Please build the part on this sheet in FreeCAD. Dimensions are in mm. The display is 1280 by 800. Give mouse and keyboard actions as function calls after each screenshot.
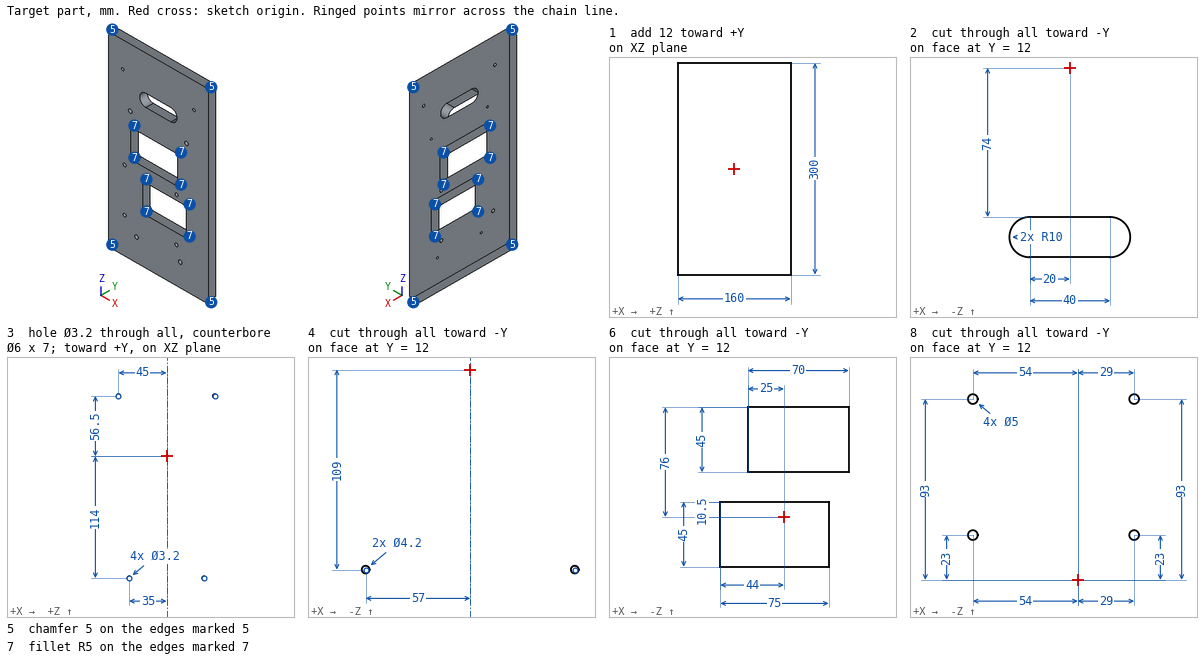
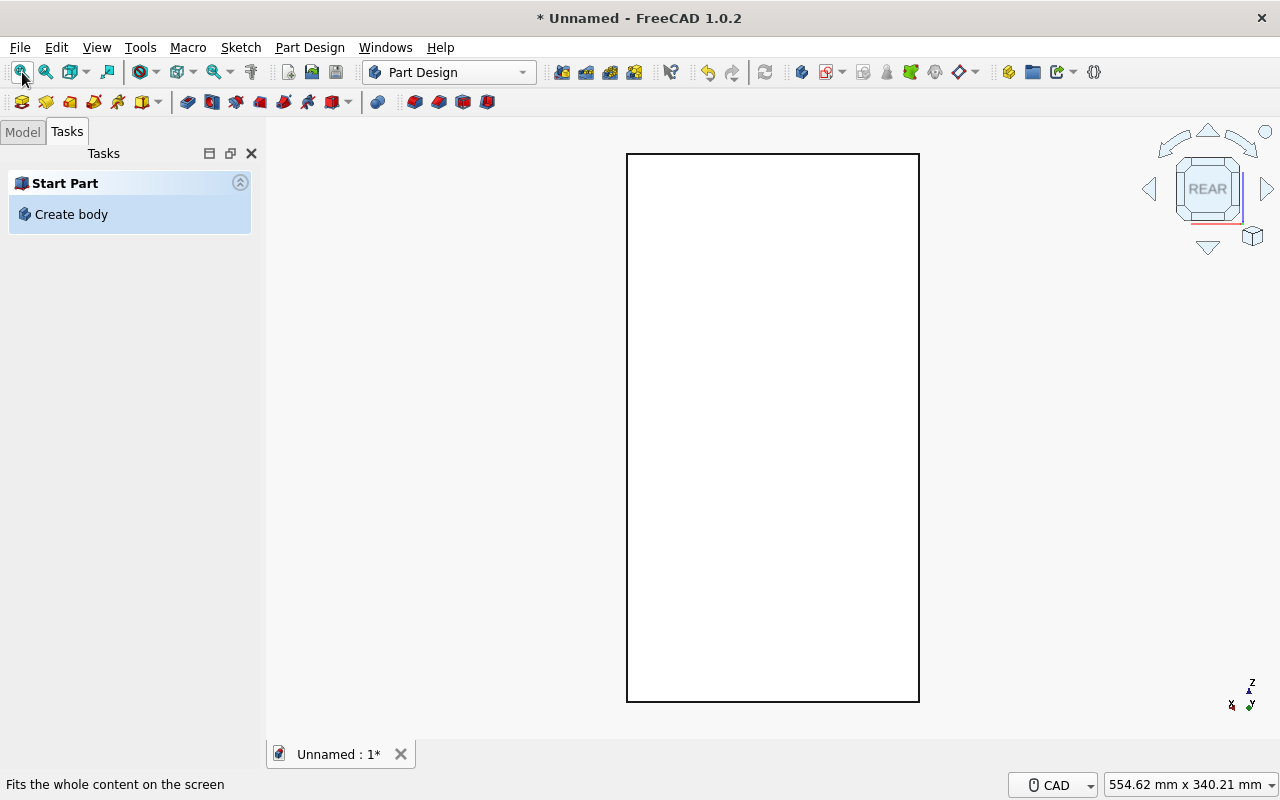
click(773, 349)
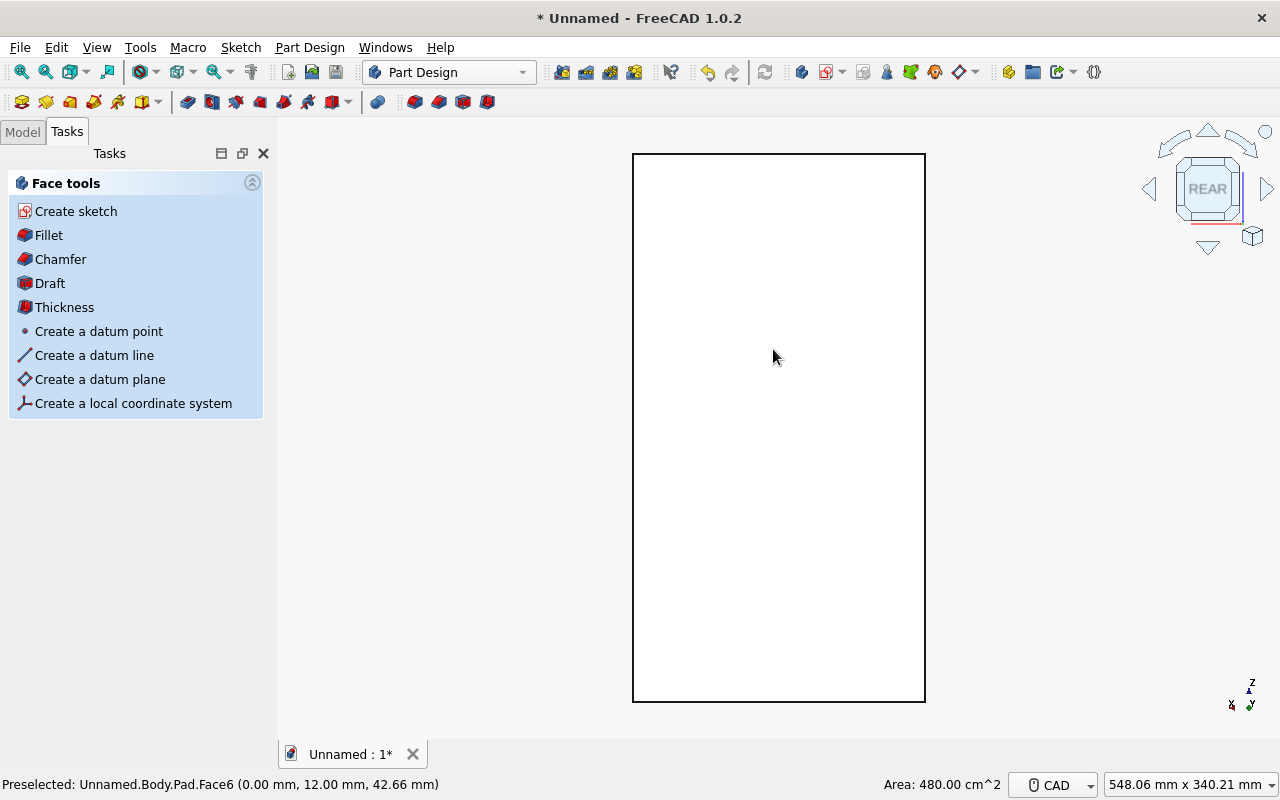
click(826, 72)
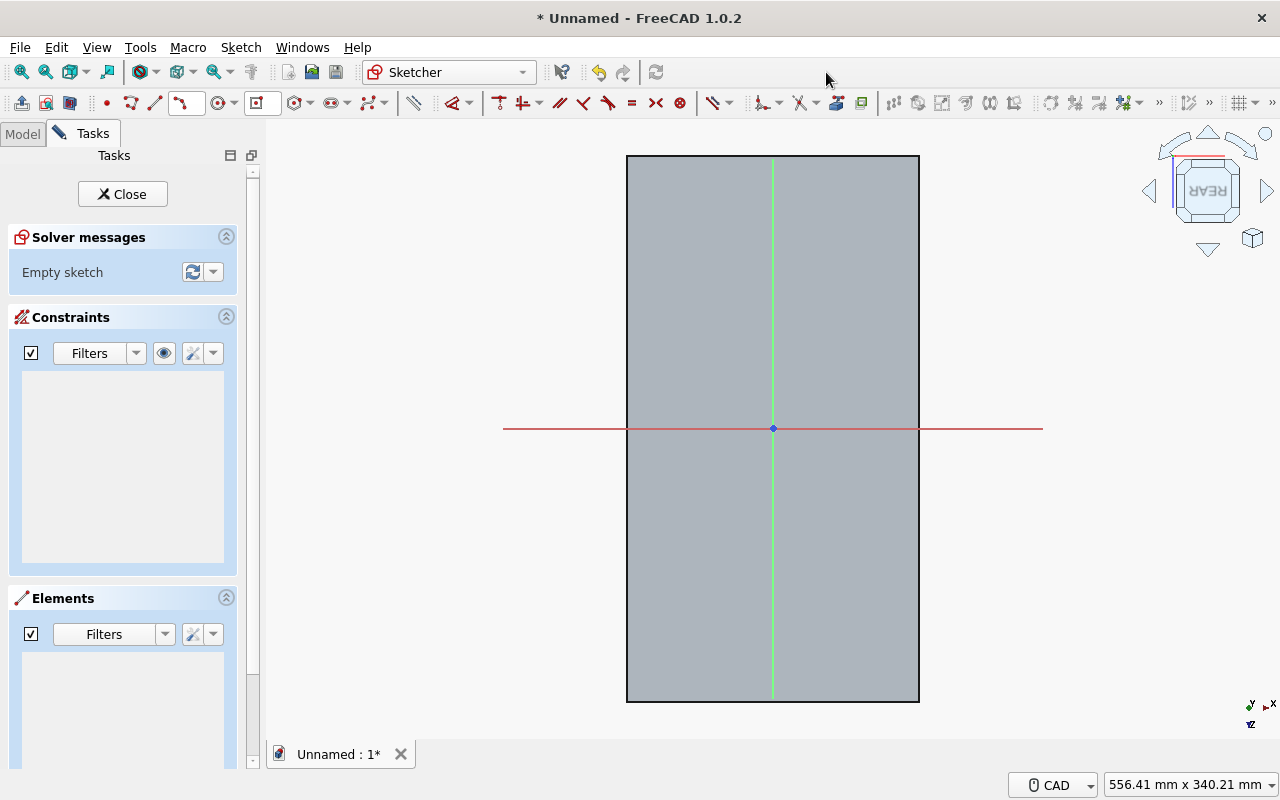
scroll(829, 585, up, 4)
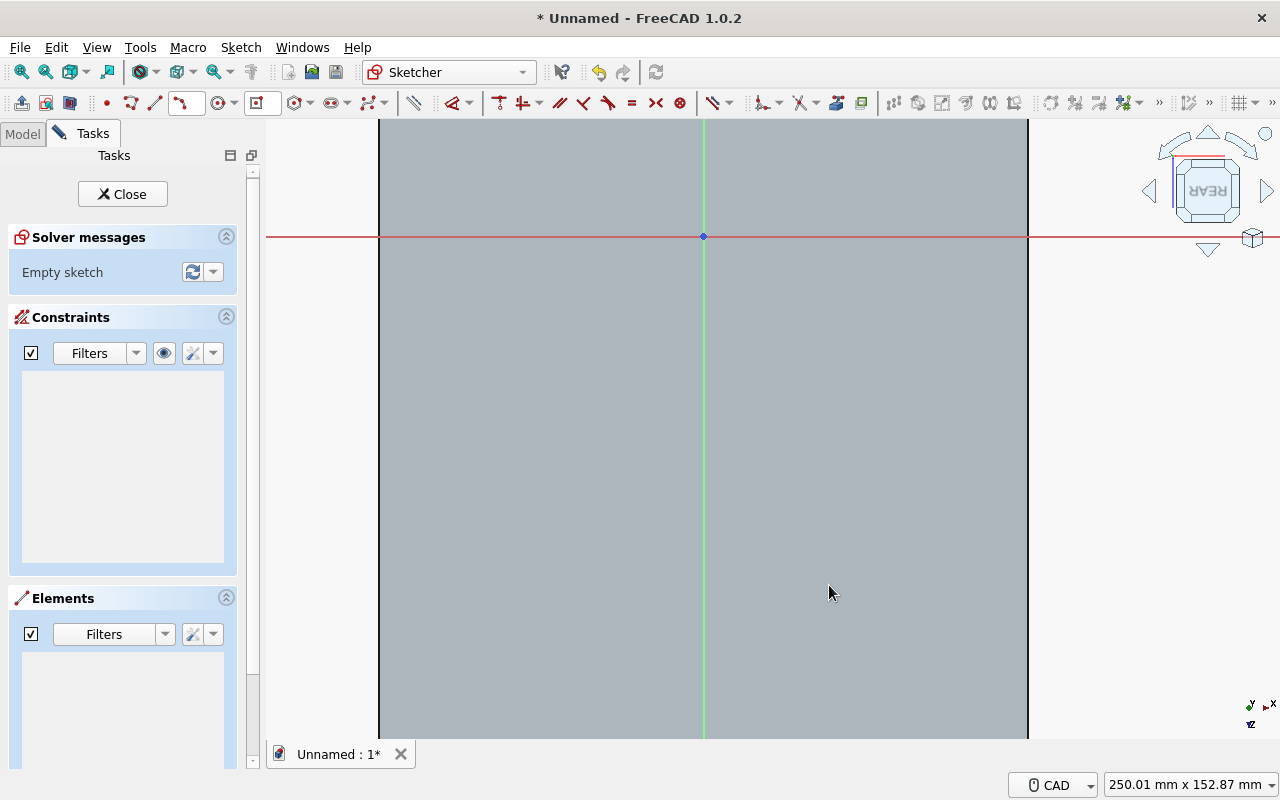
click(332, 104)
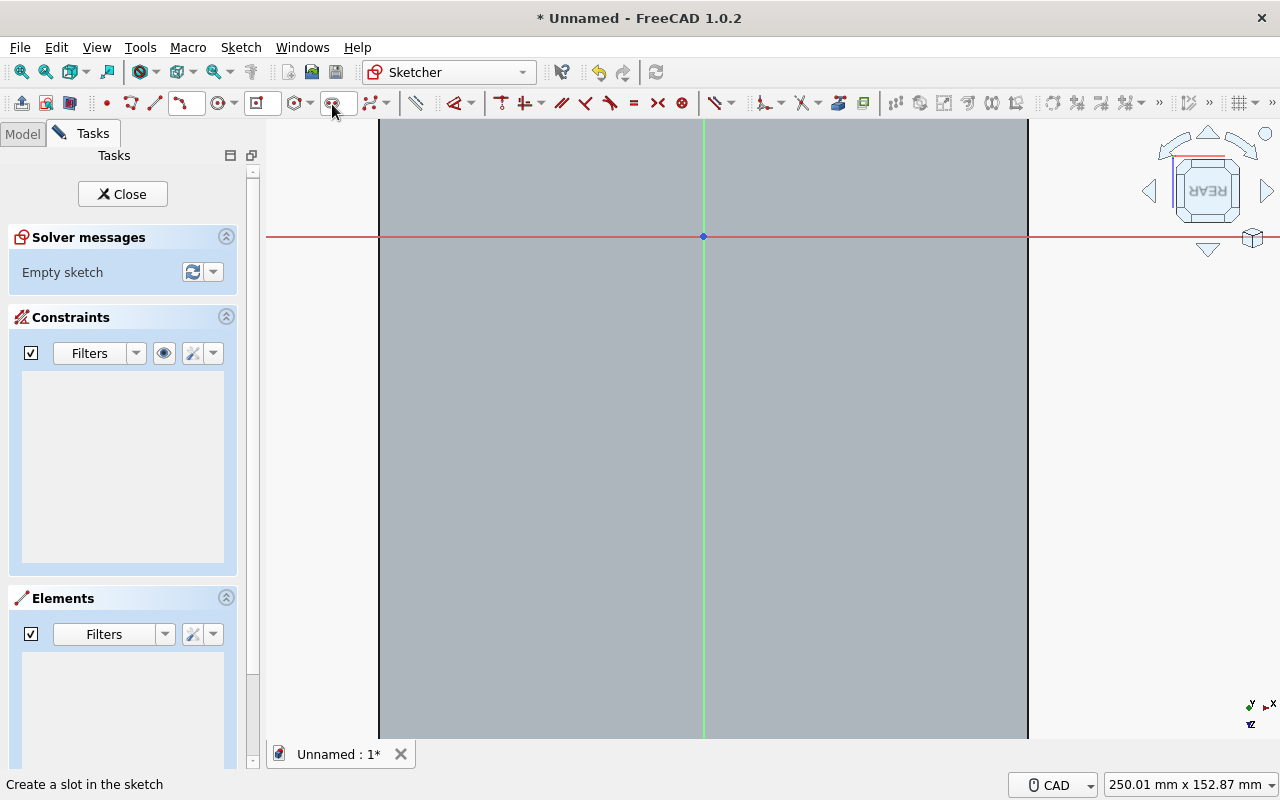
click(623, 578)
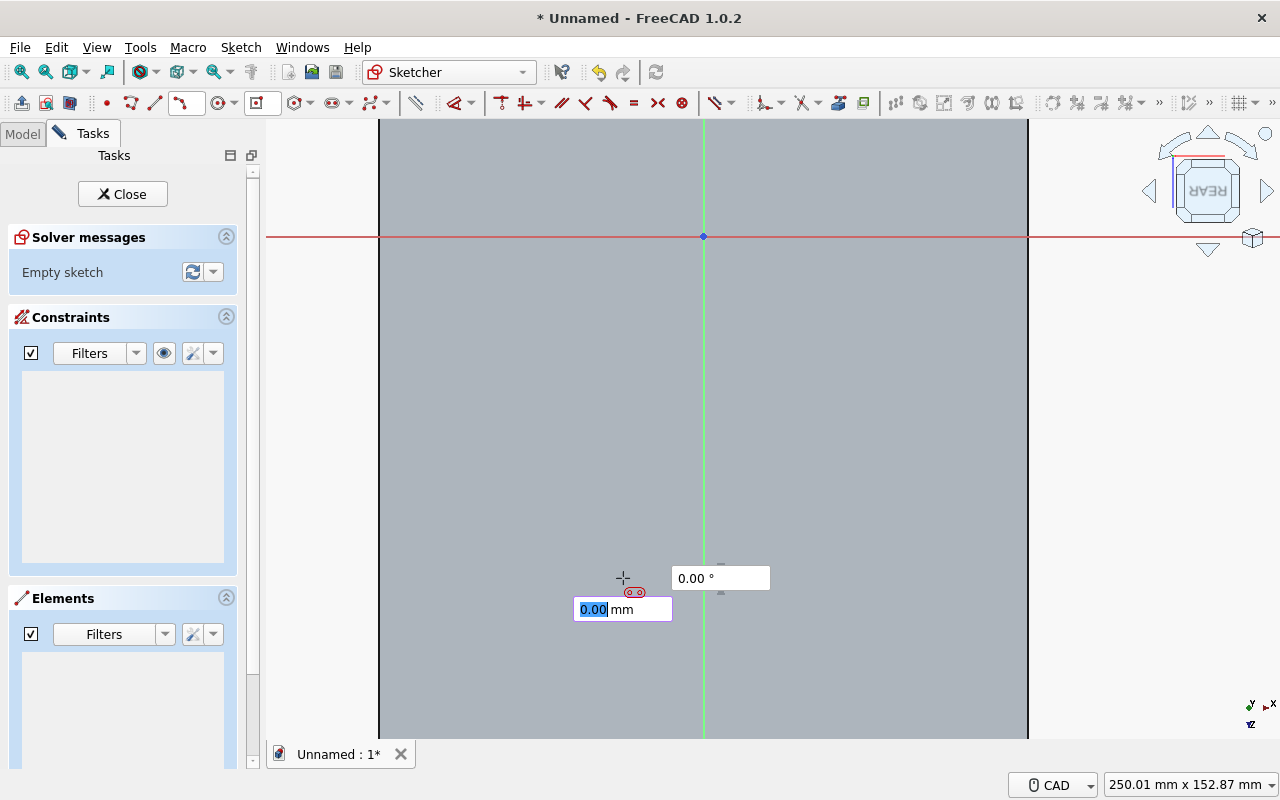
click(785, 578)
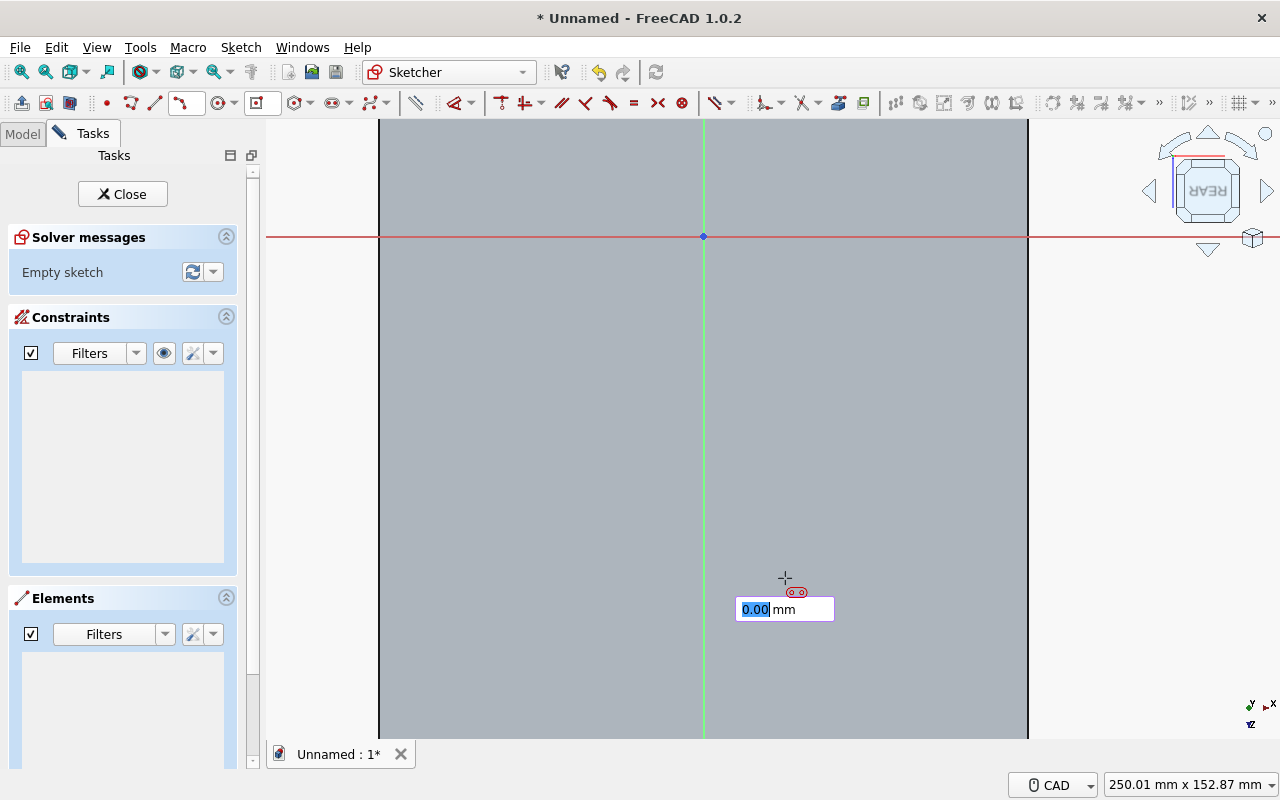
click(728, 537)
key(Escape)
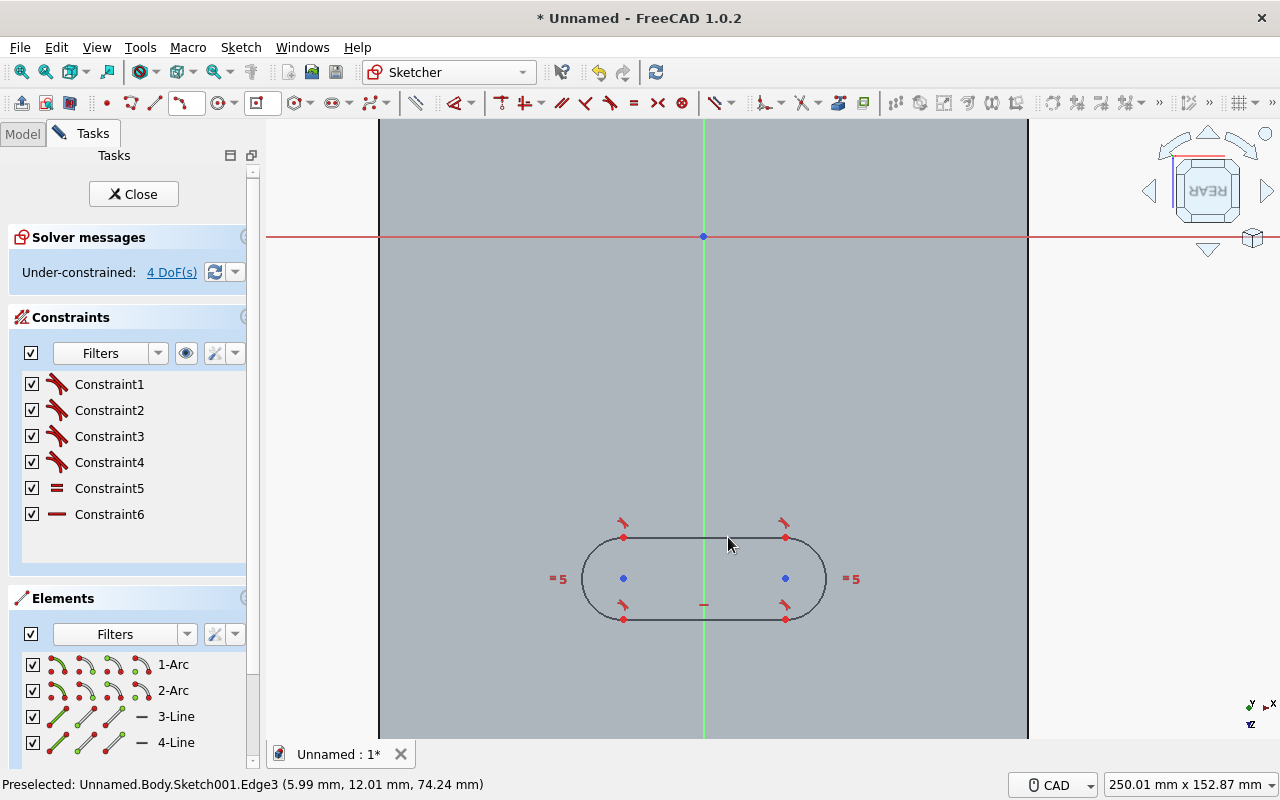
click(454, 104)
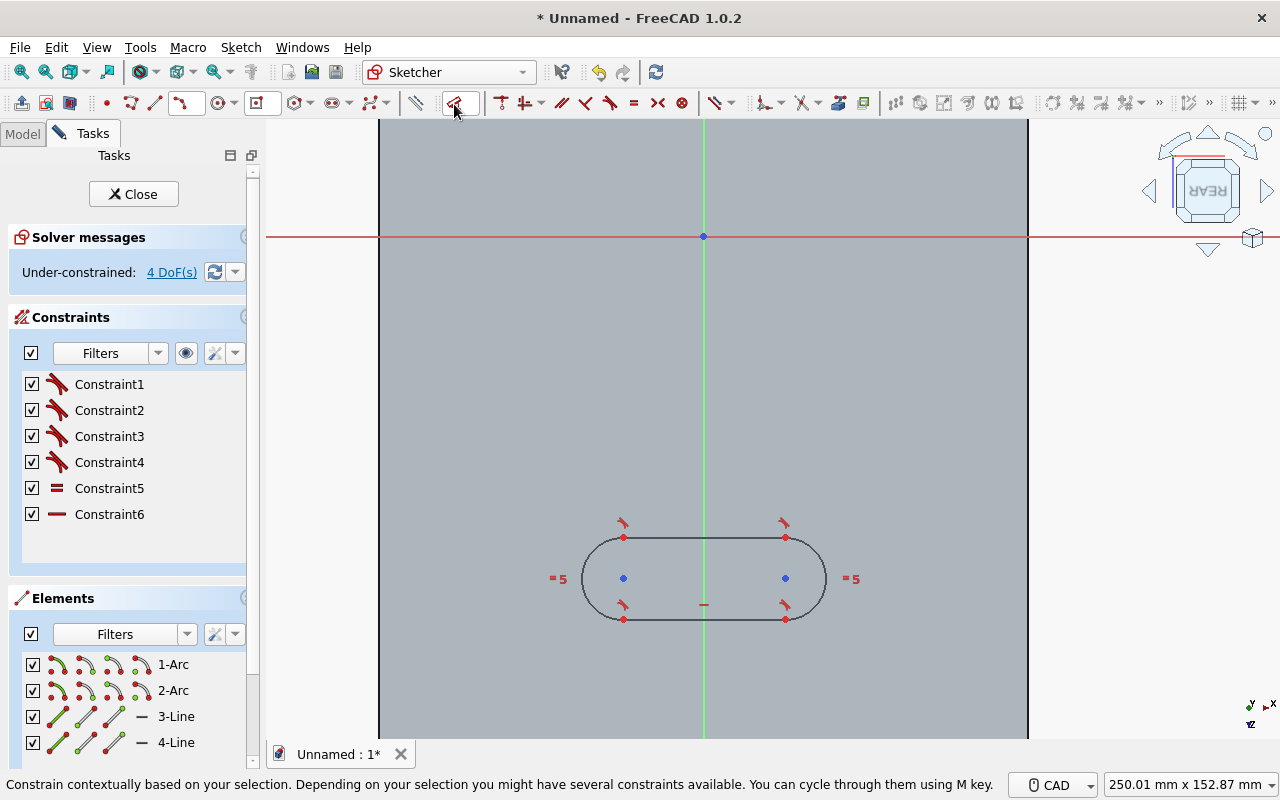
click(590, 555)
click(564, 536)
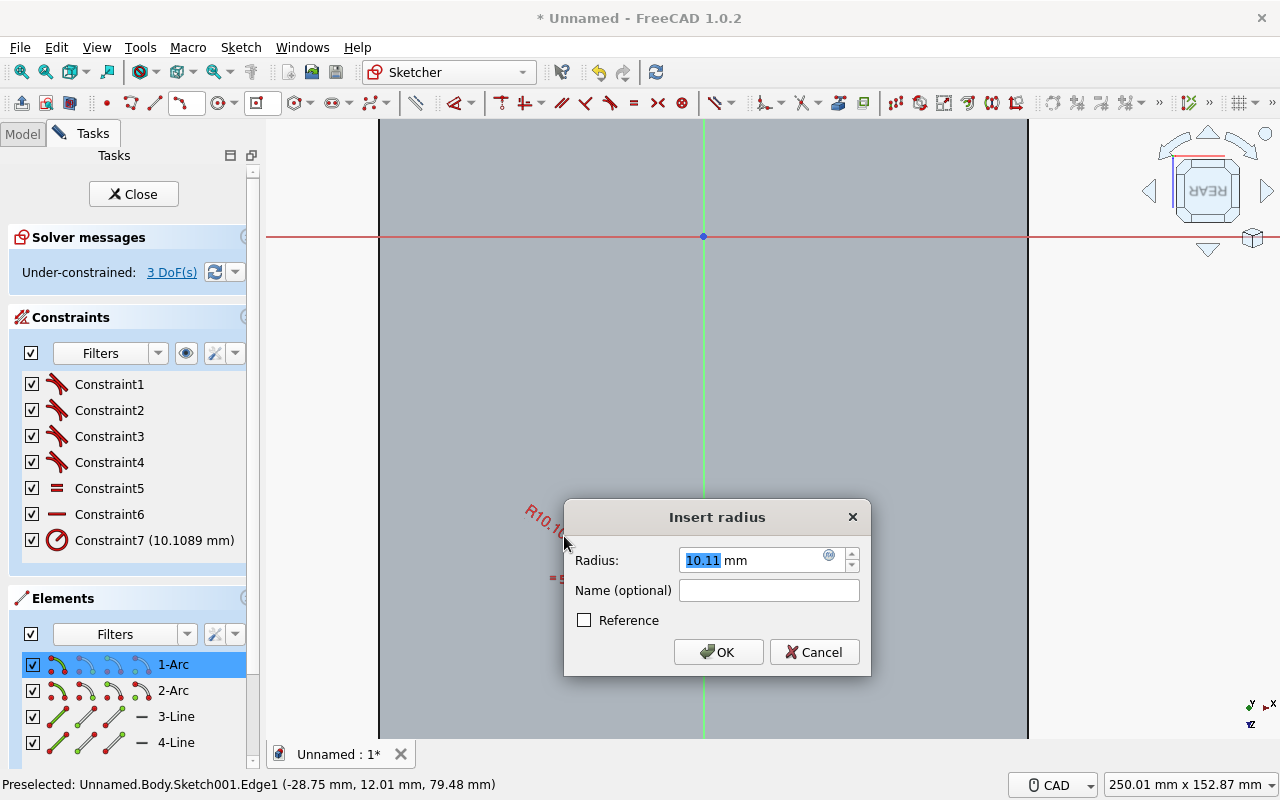
text(10)
key(Return)